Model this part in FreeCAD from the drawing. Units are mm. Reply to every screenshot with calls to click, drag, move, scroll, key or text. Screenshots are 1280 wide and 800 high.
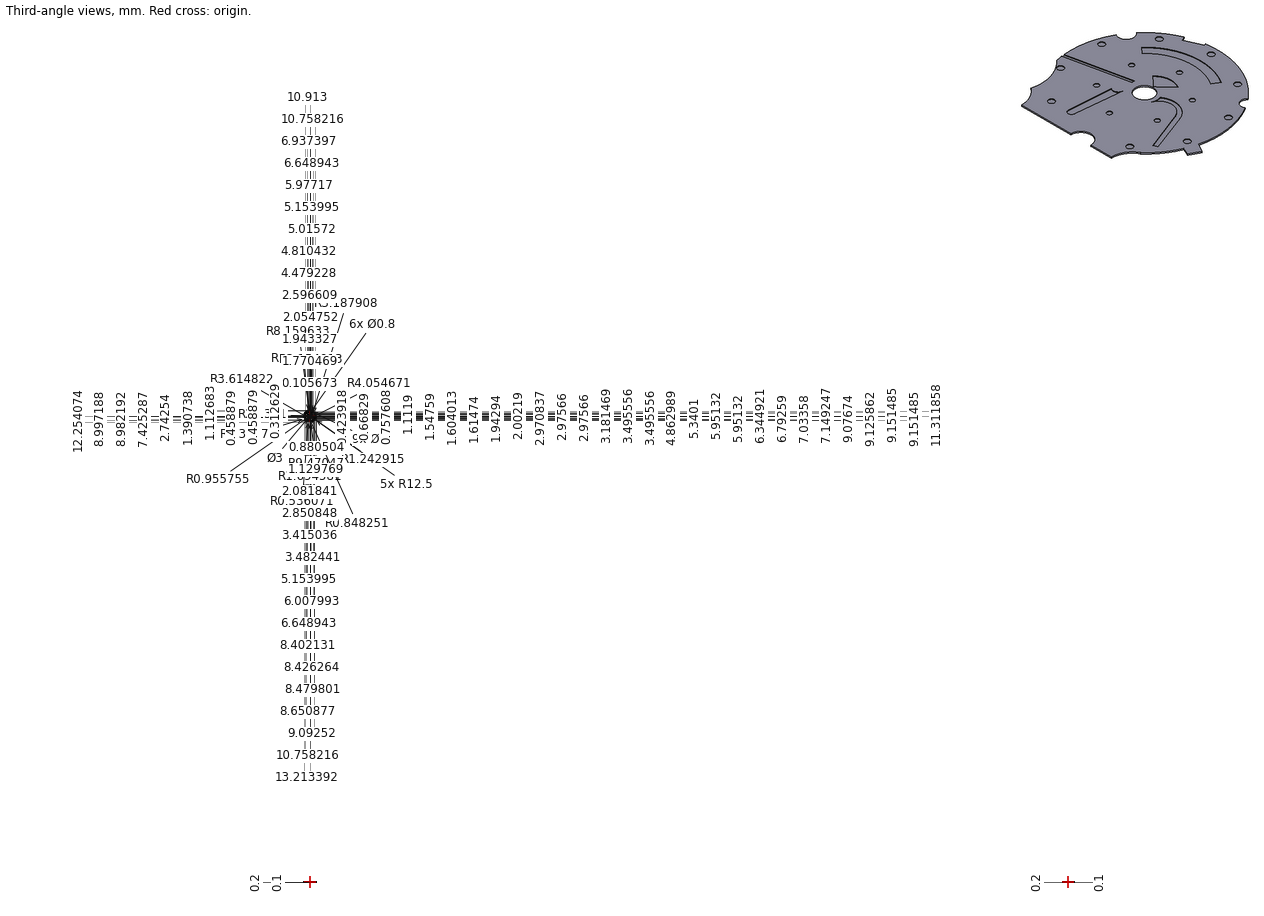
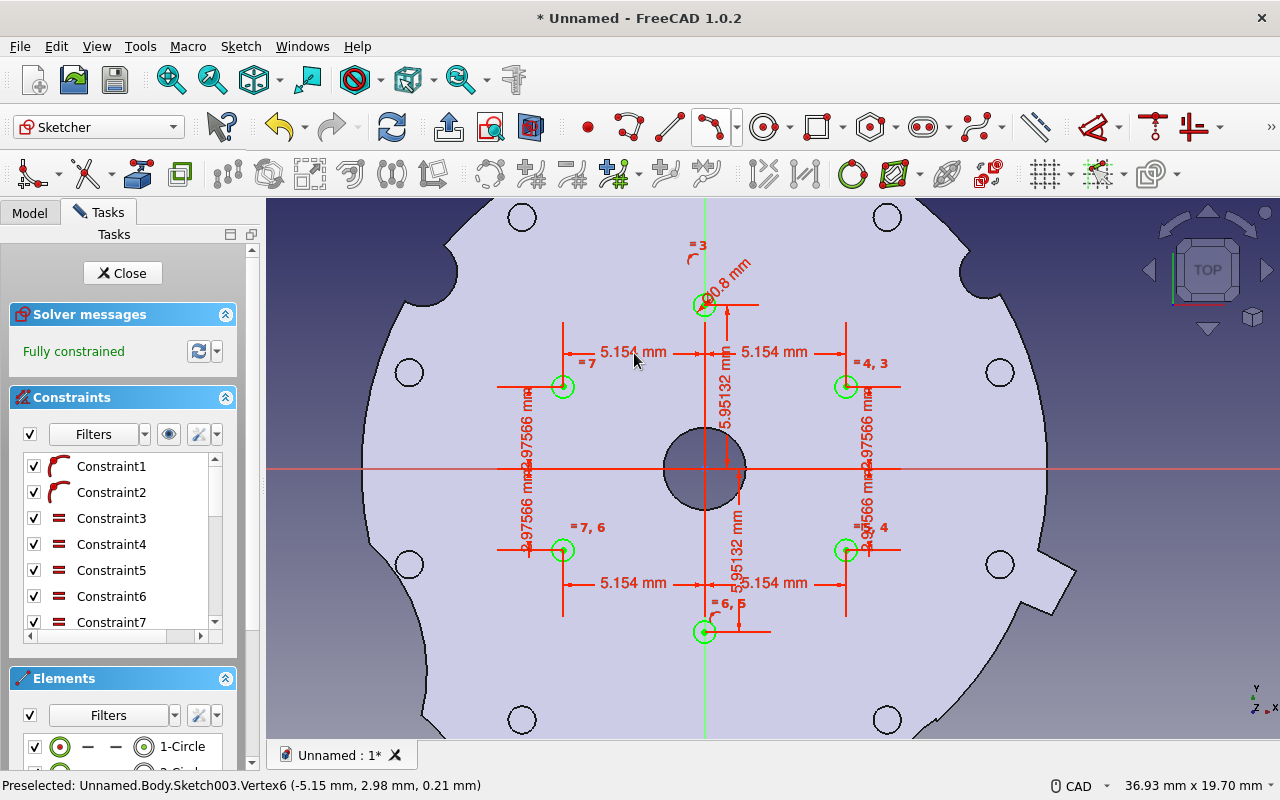
click(123, 273)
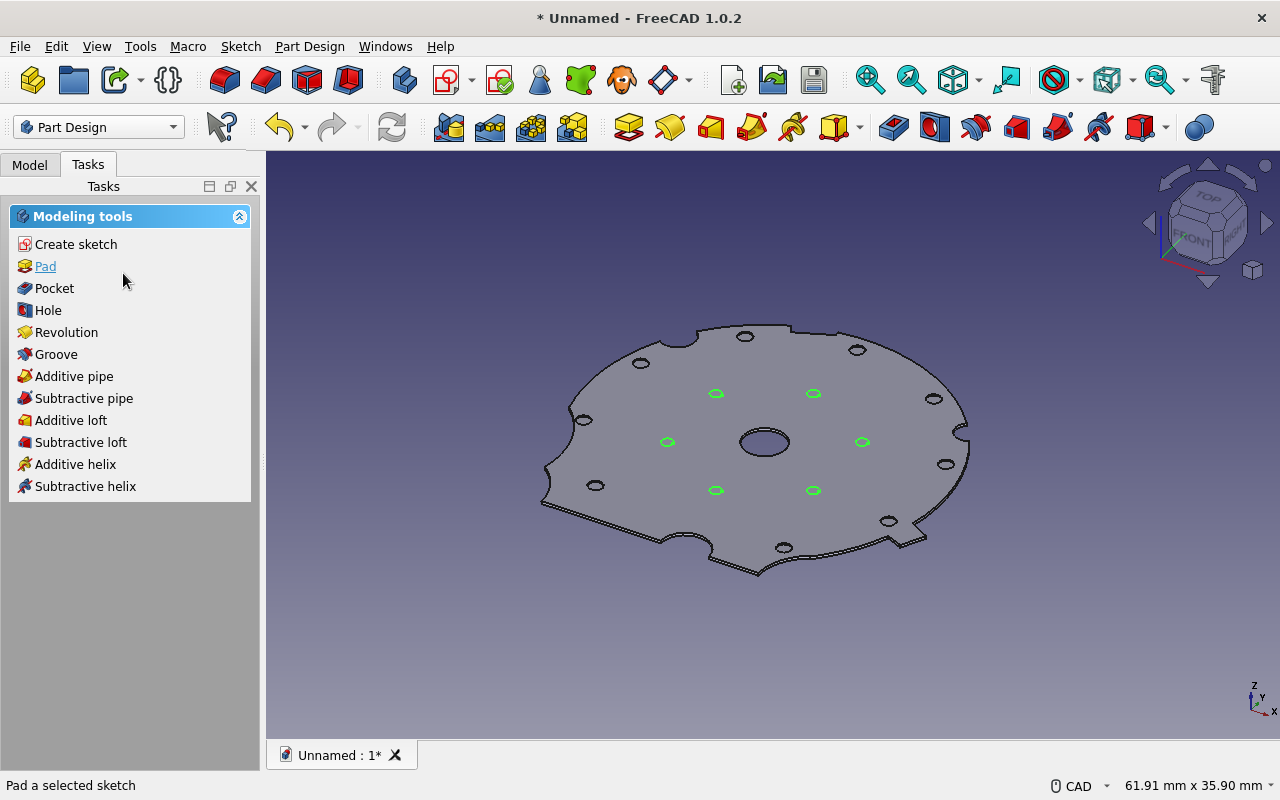
click(894, 128)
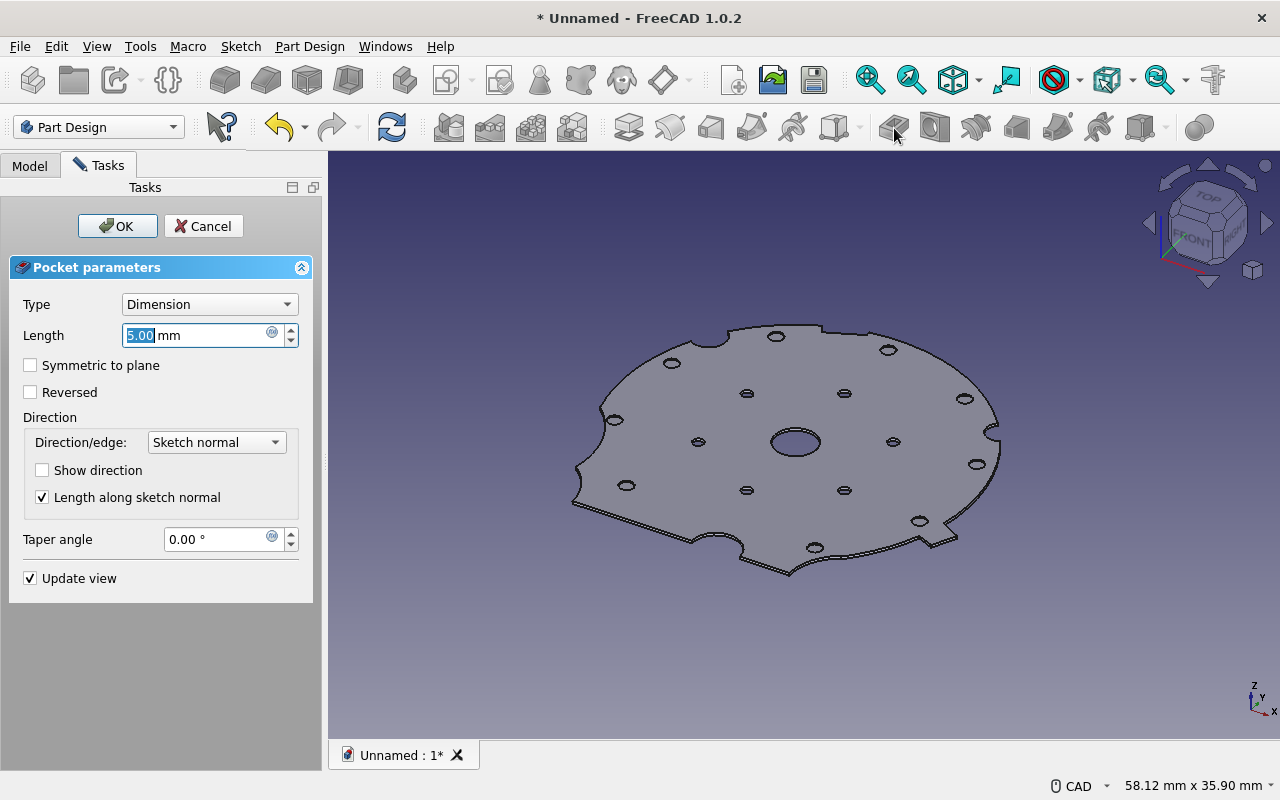
text(0.1)
key(Tab)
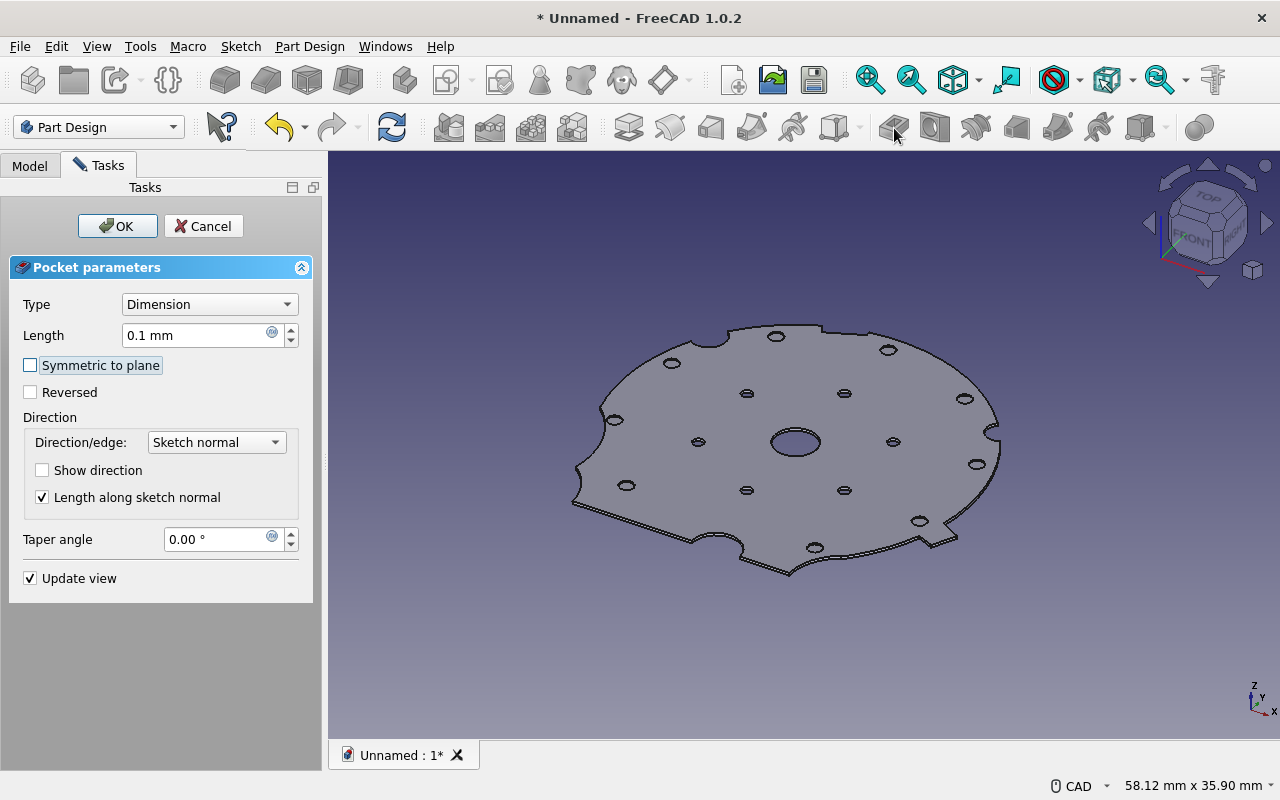
click(118, 226)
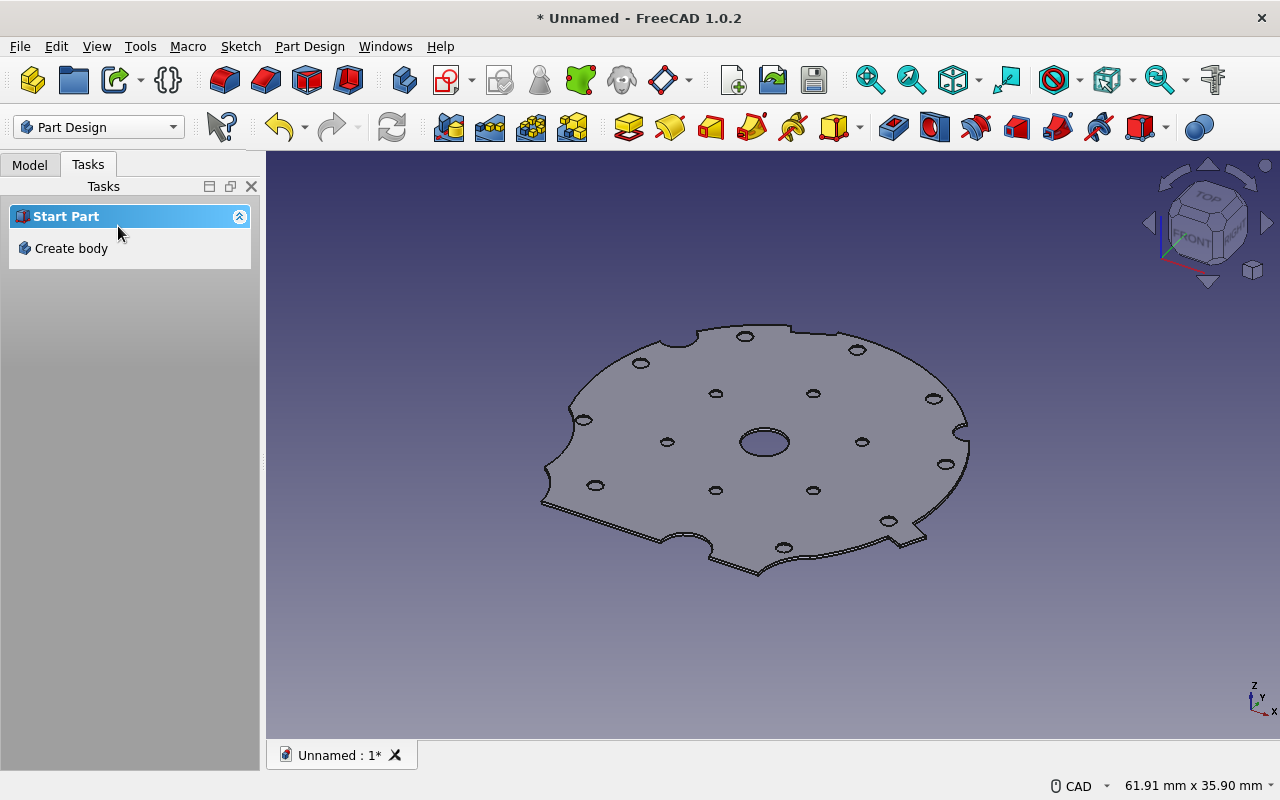
click(878, 477)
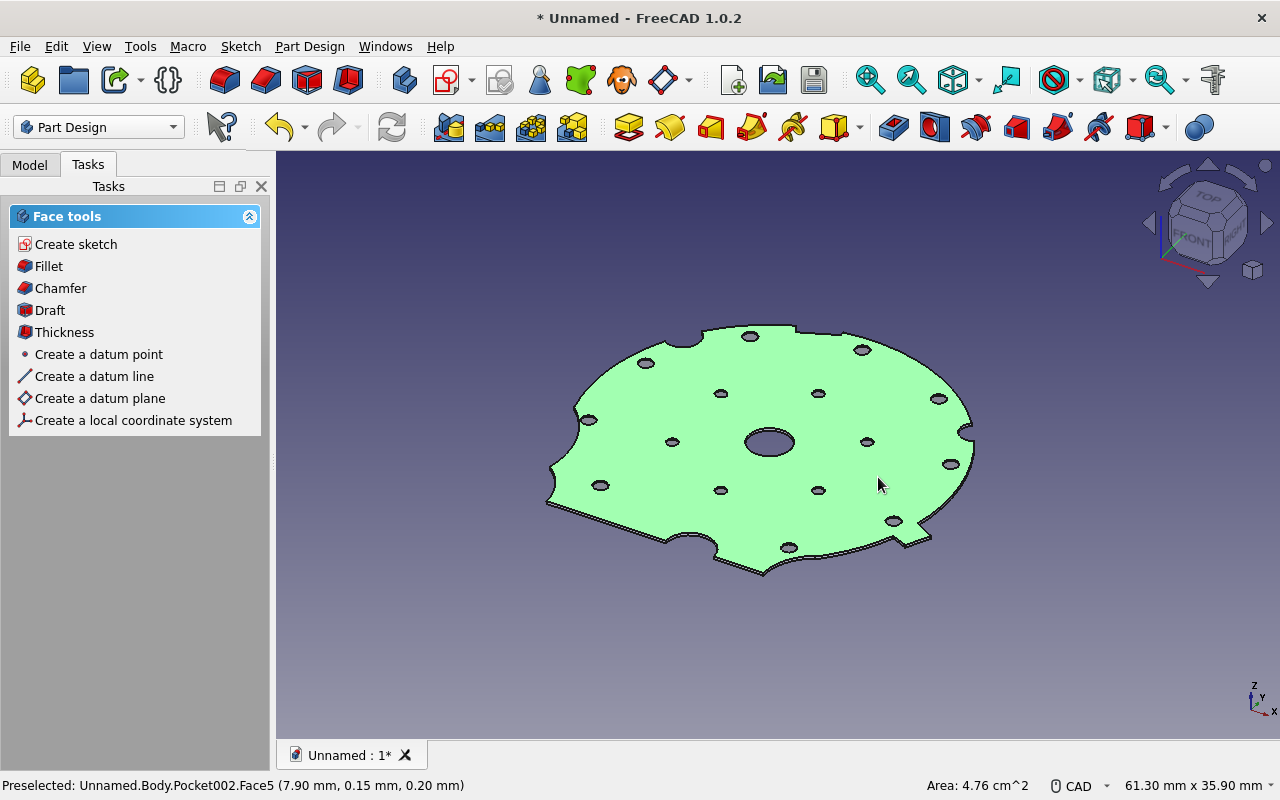
click(446, 80)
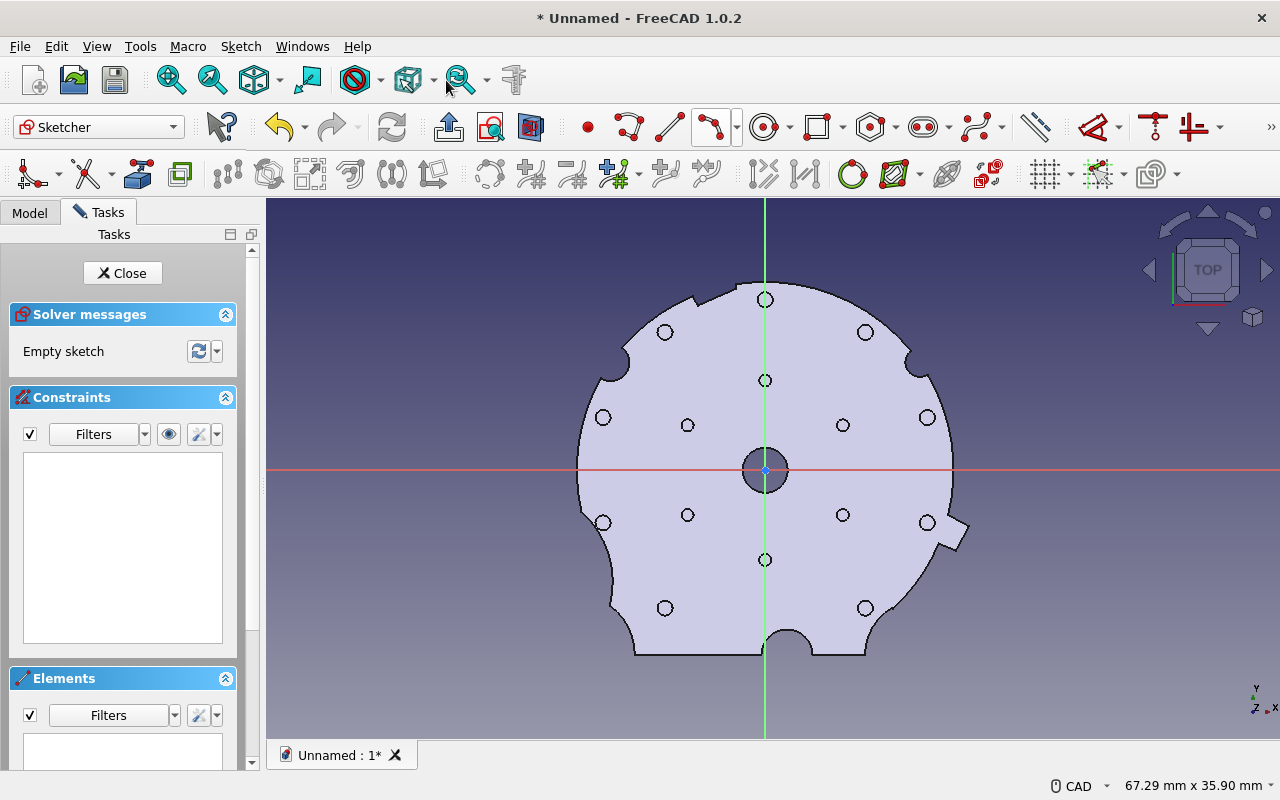
key(g)
key(l)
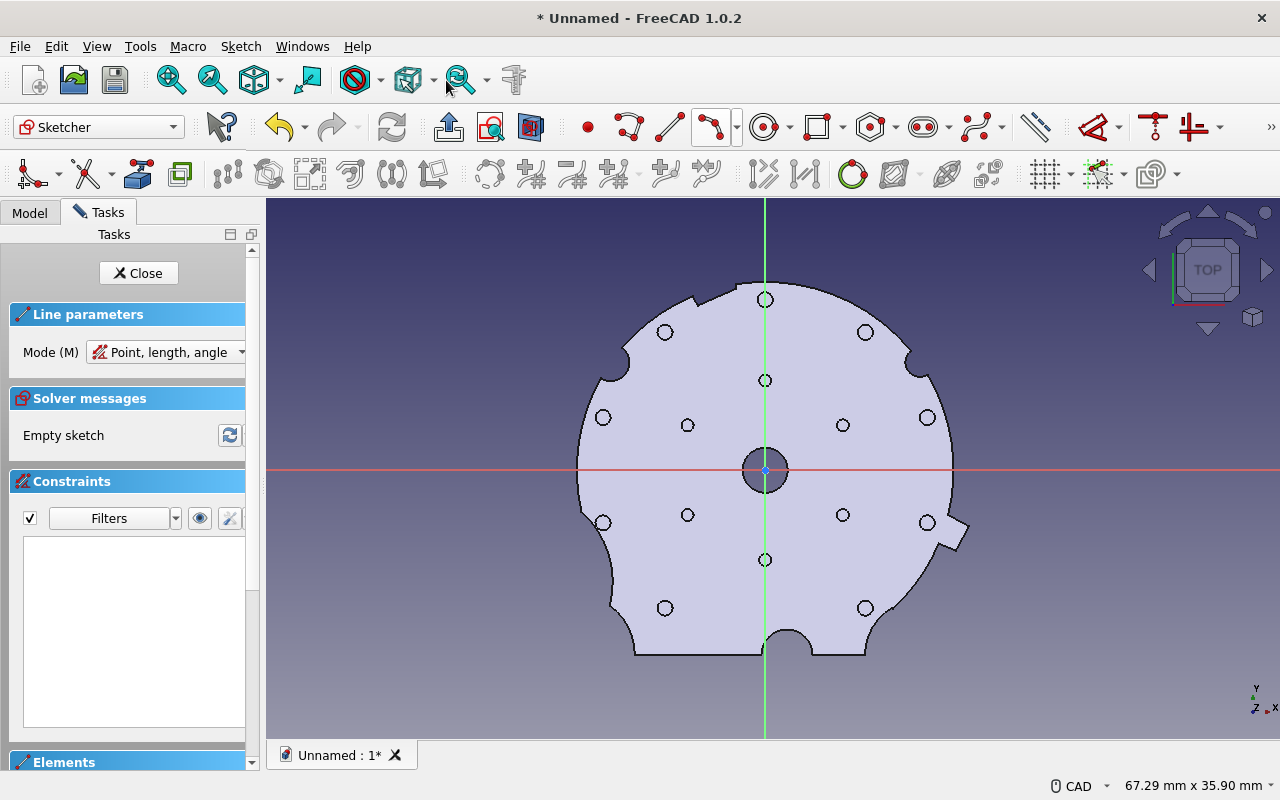
click(661, 373)
click(675, 387)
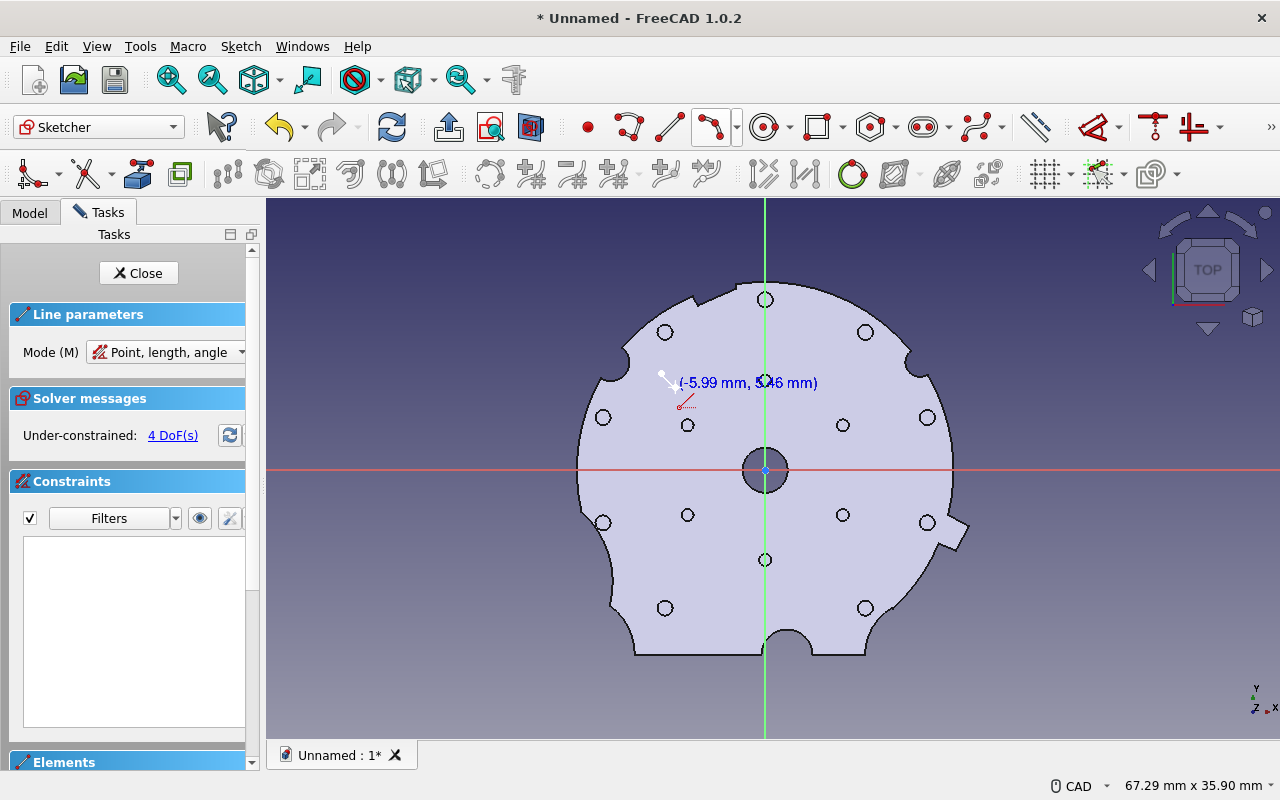
click(830, 366)
click(841, 349)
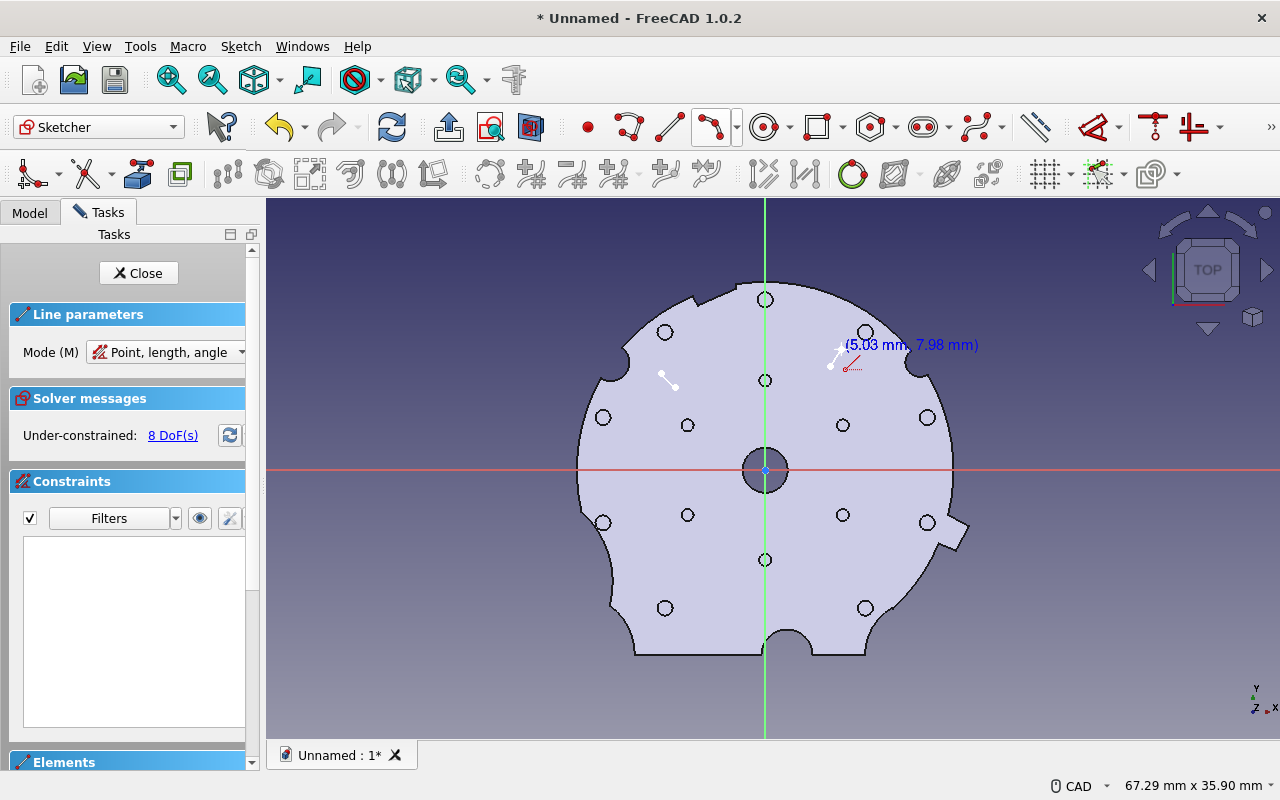
key(g)
key(3)
key(a)